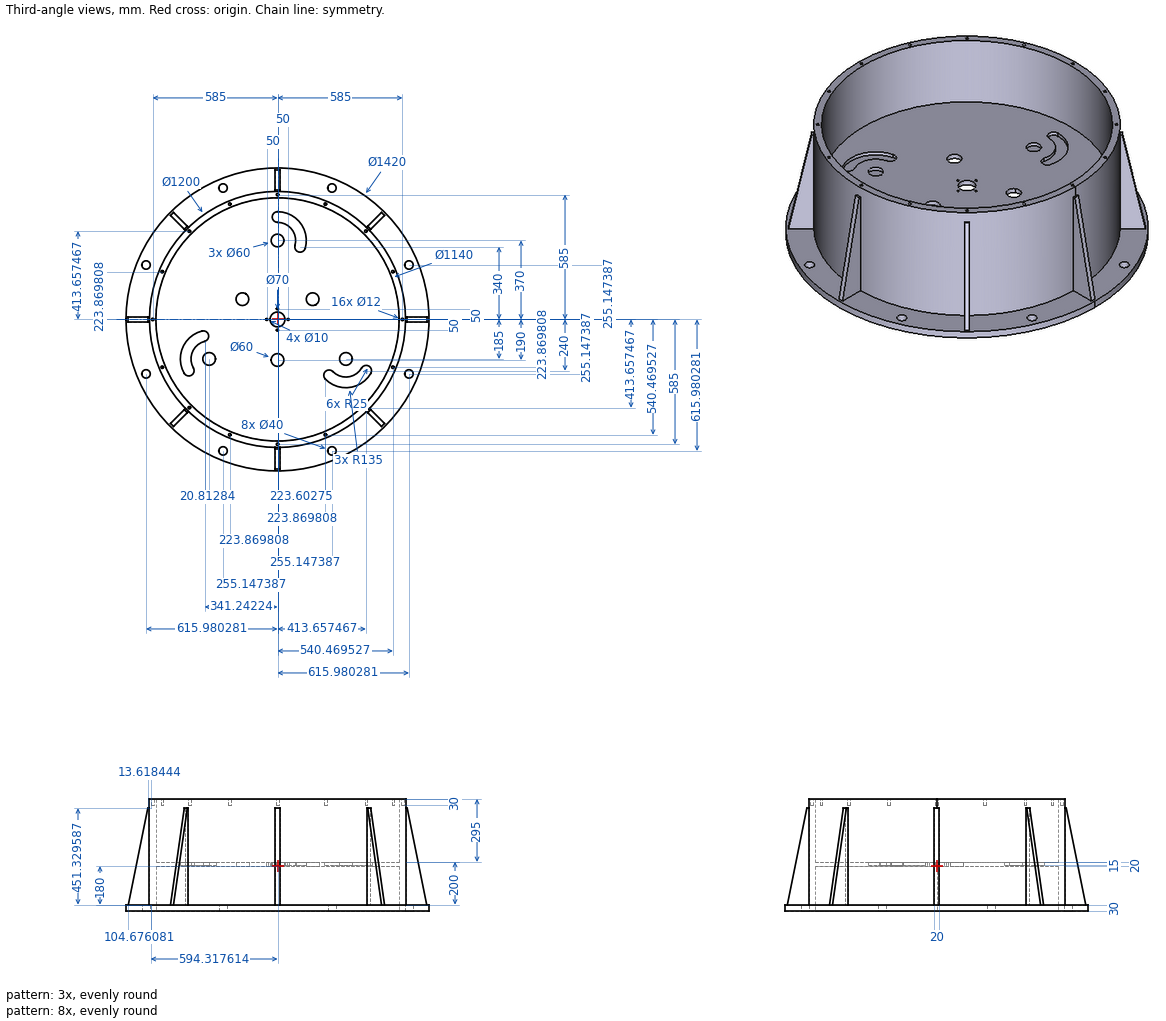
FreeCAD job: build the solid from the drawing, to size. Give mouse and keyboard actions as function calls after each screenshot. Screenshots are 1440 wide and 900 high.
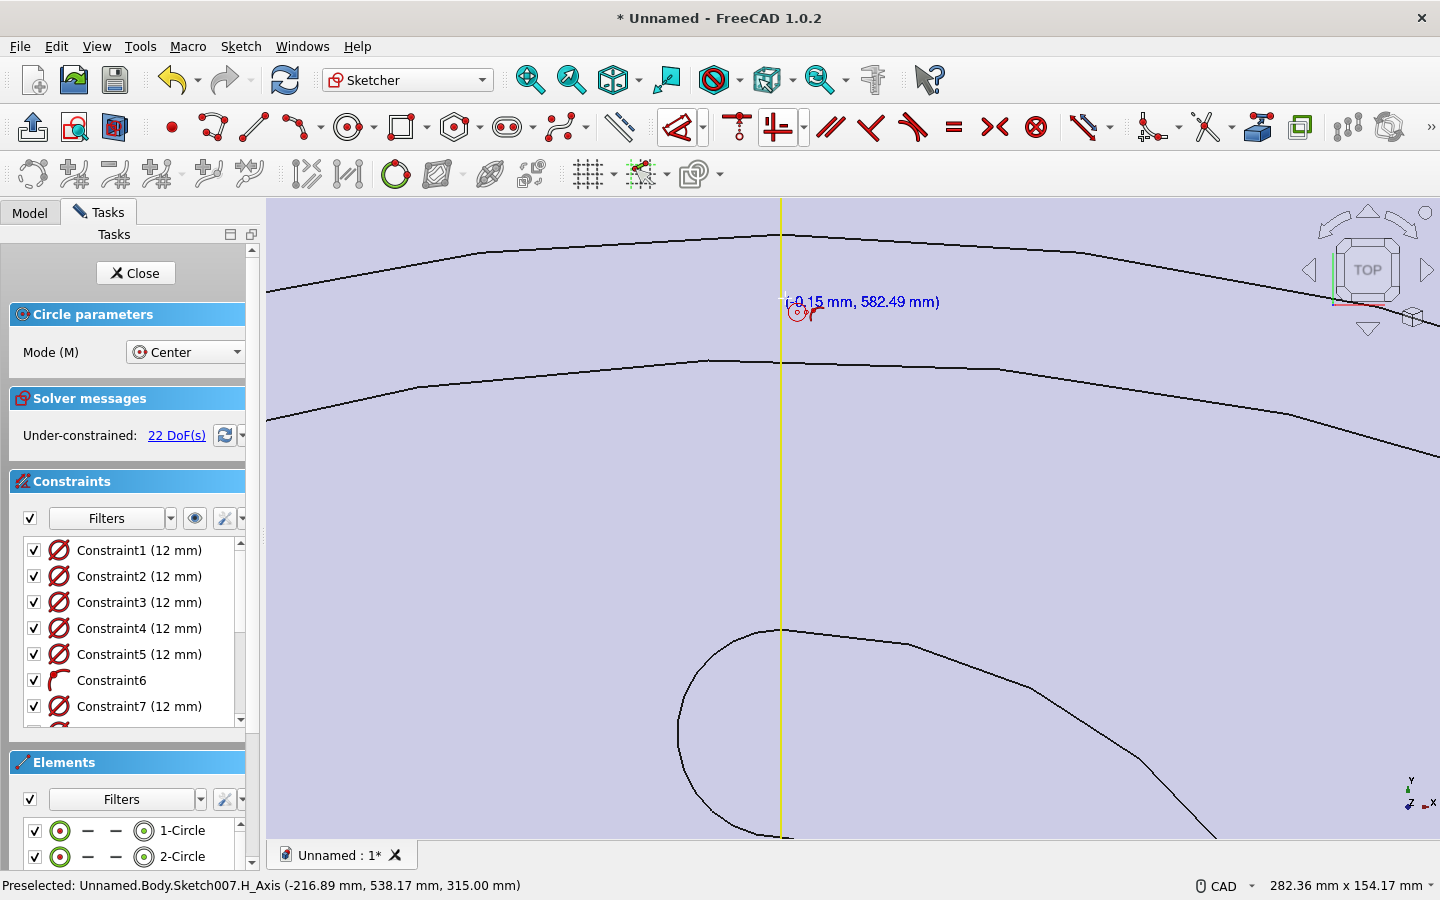
scroll(785, 298, down, 12)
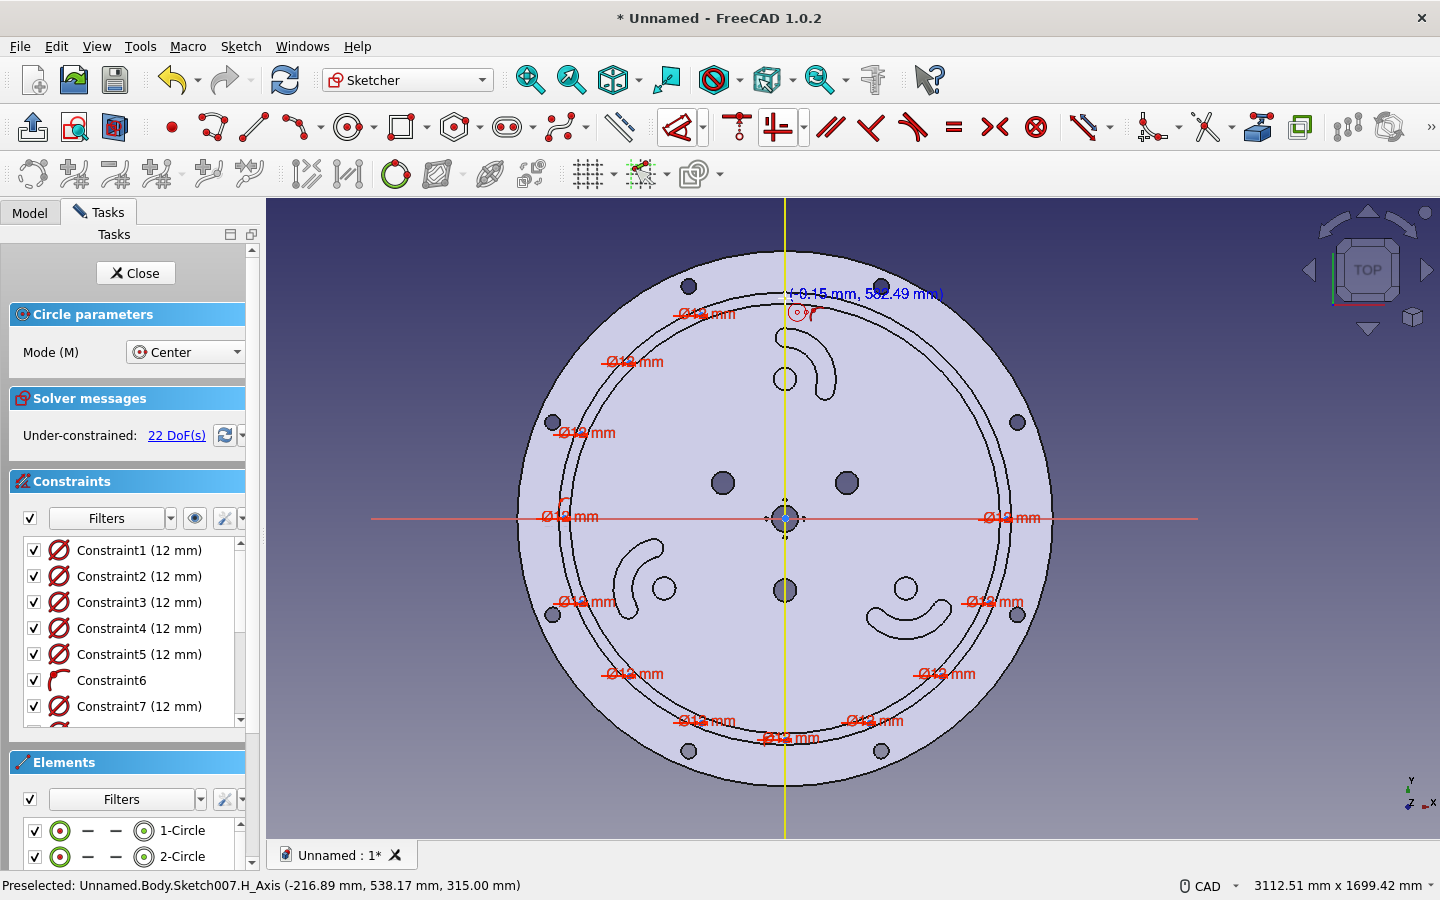
click(785, 298)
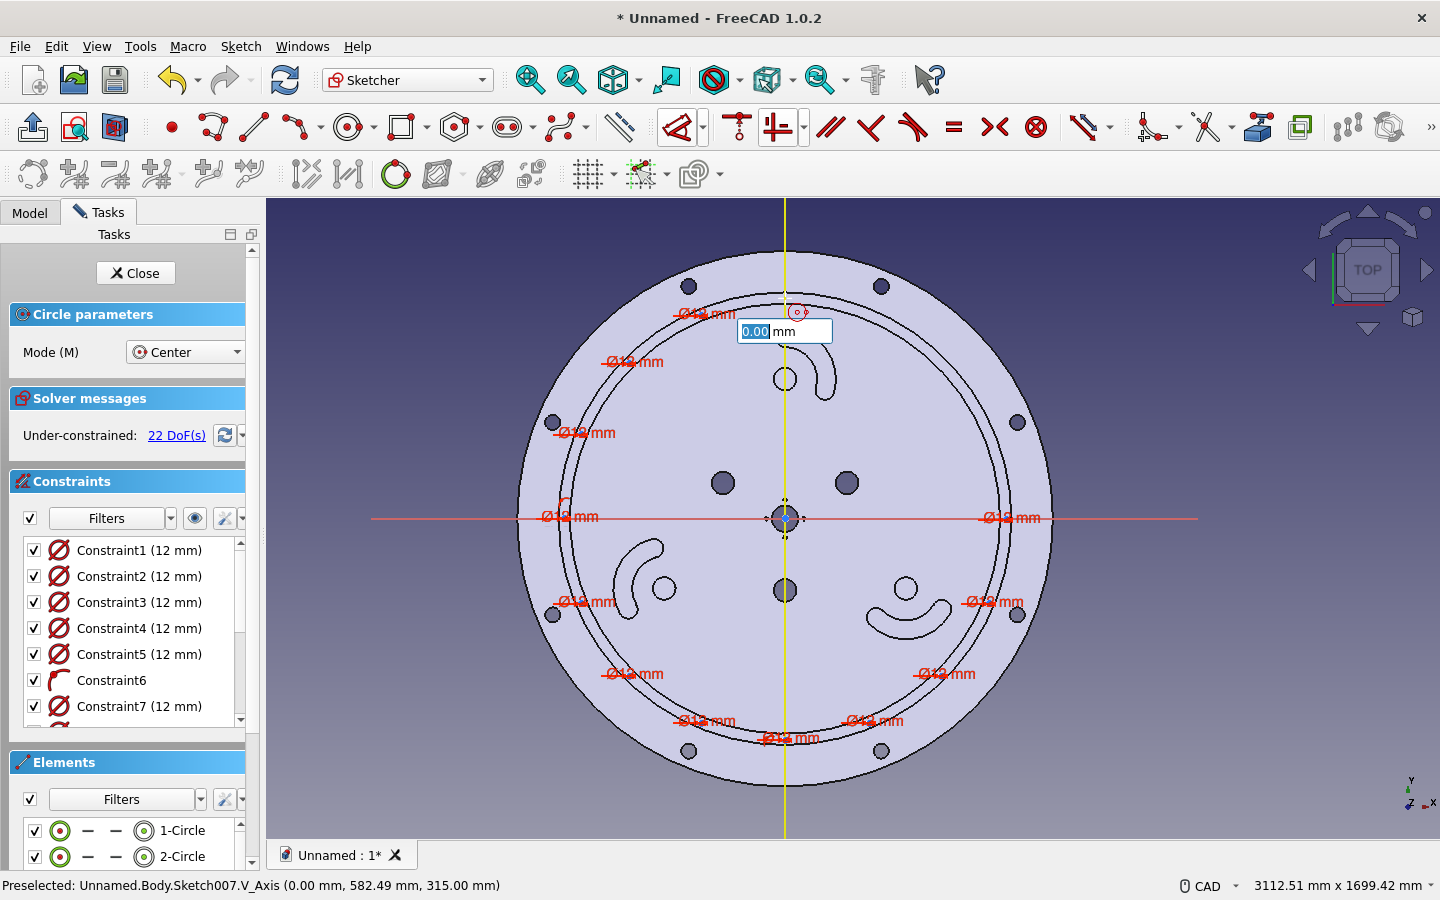
scroll(787, 297, up, 11)
move(785, 298)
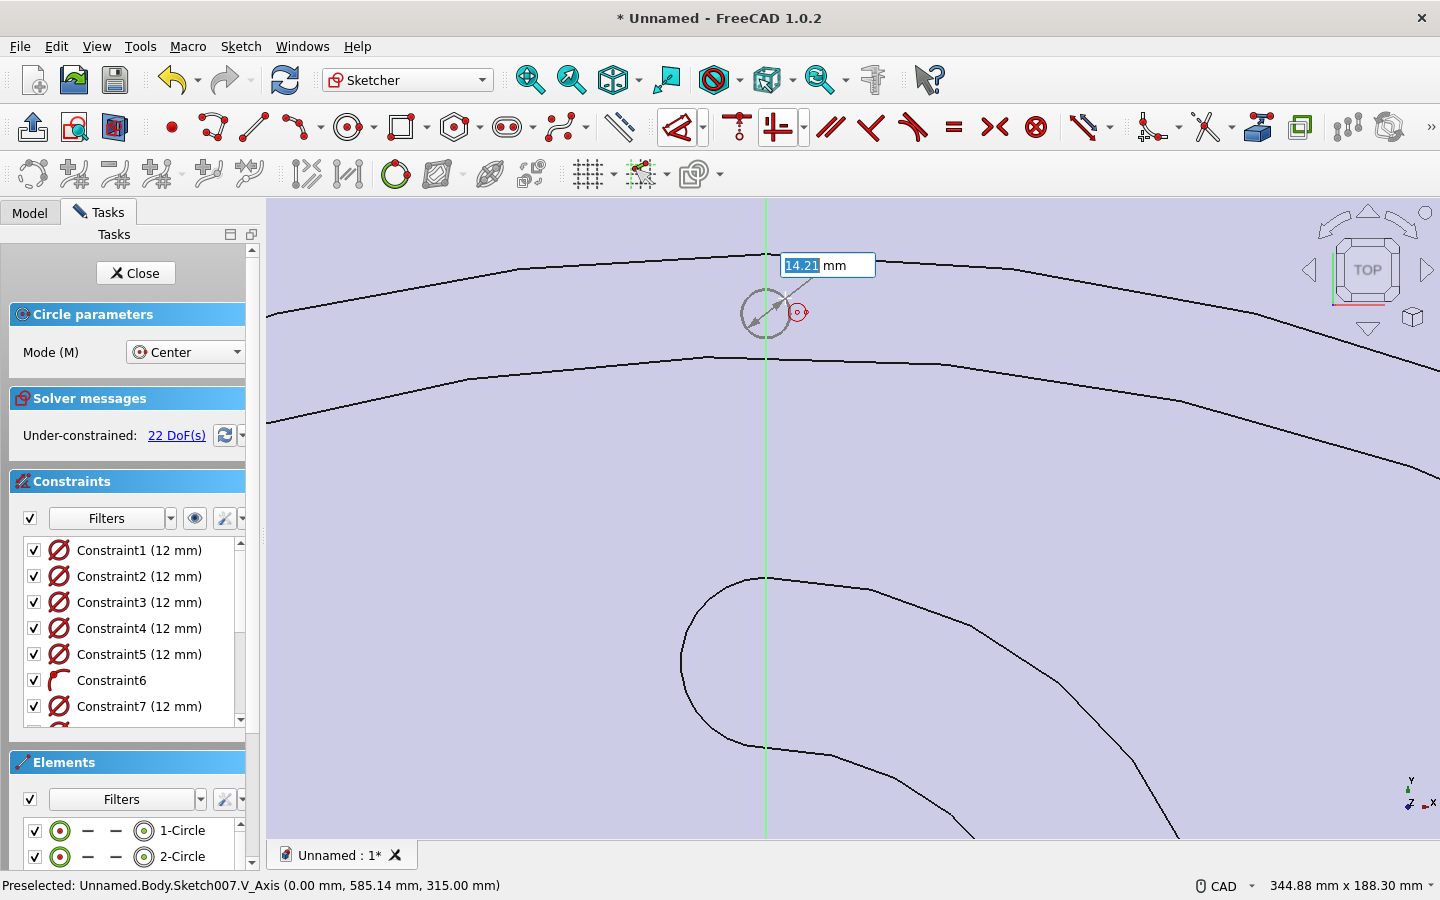
text(12)
key(Return)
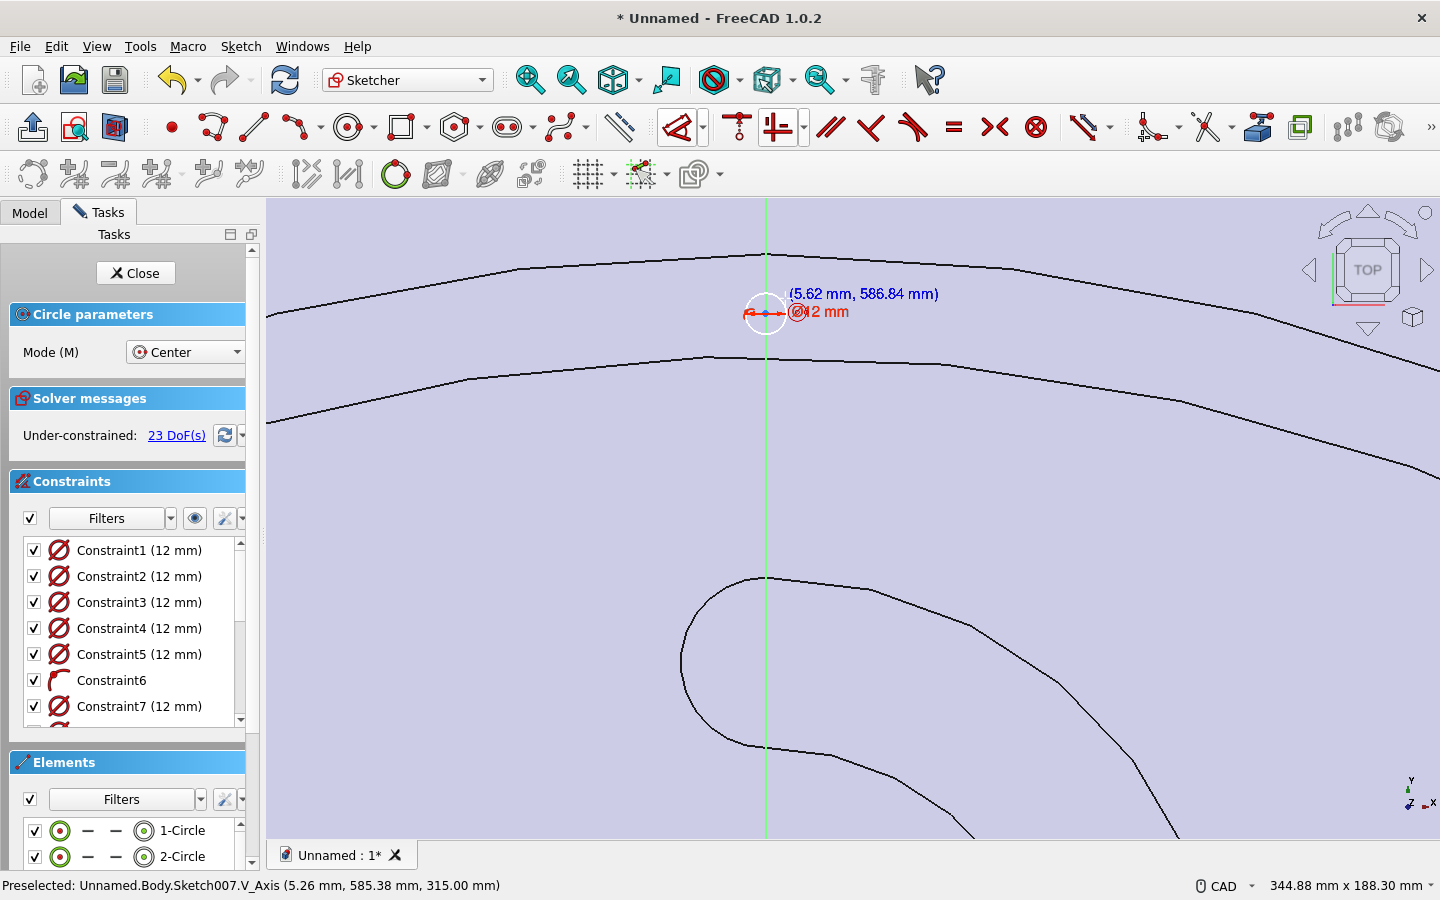
scroll(787, 297, down, 11)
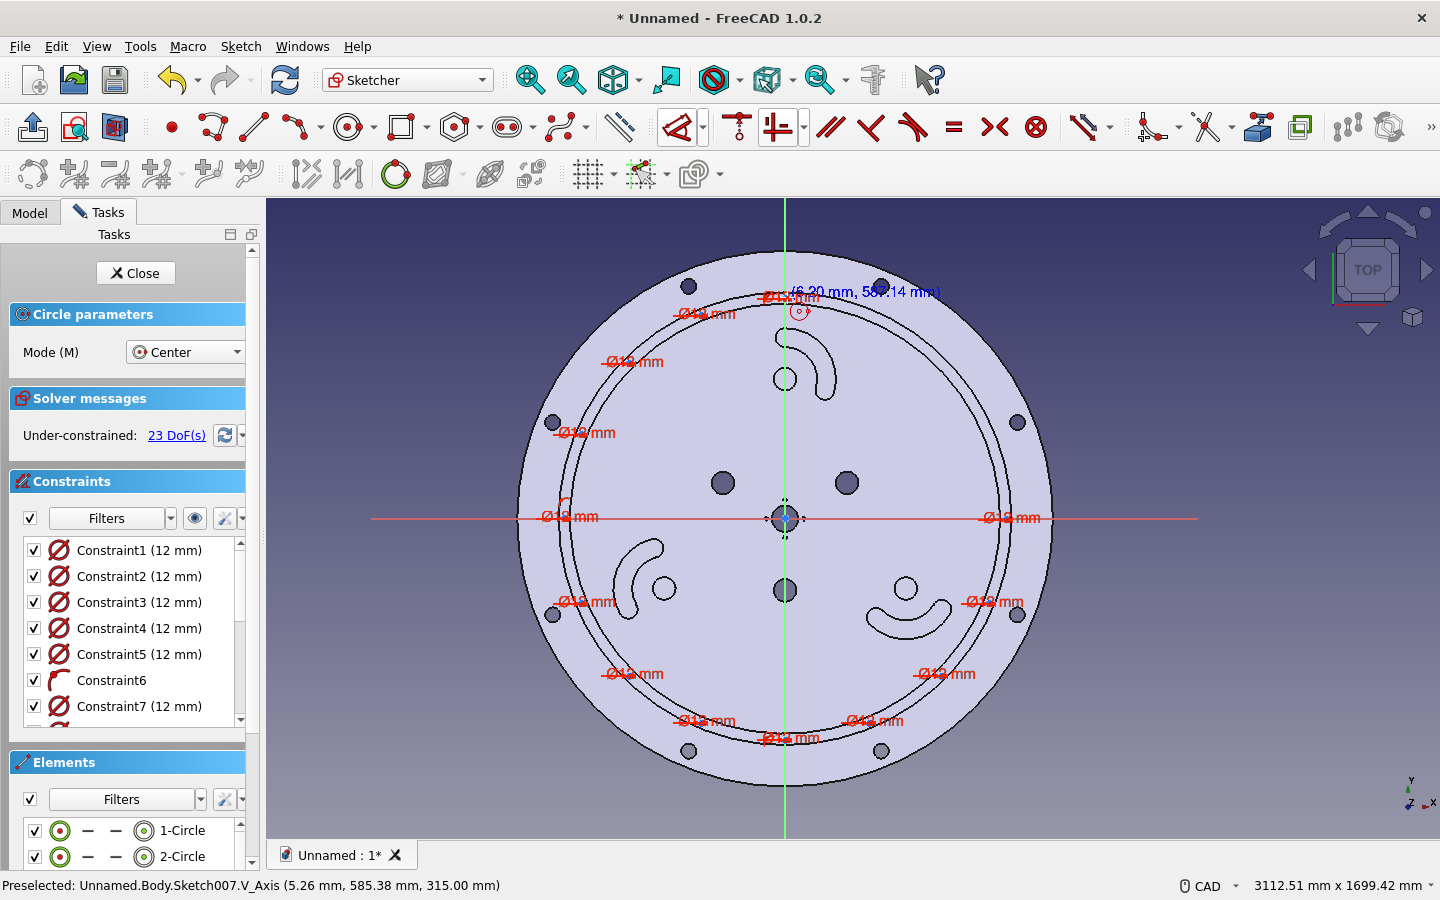
scroll(869, 315, up, 12)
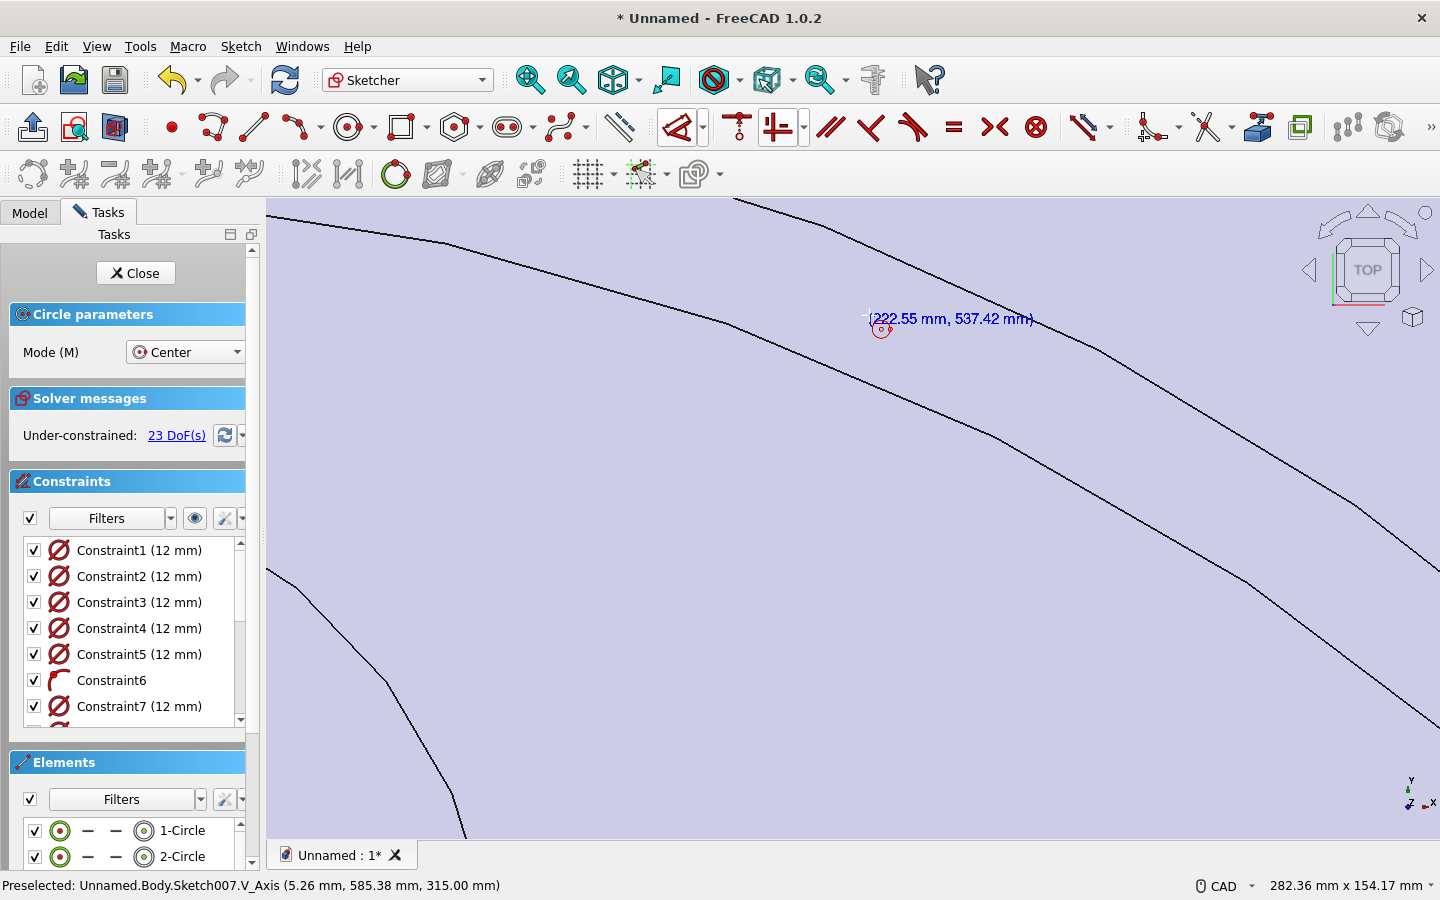
scroll(869, 315, down, 12)